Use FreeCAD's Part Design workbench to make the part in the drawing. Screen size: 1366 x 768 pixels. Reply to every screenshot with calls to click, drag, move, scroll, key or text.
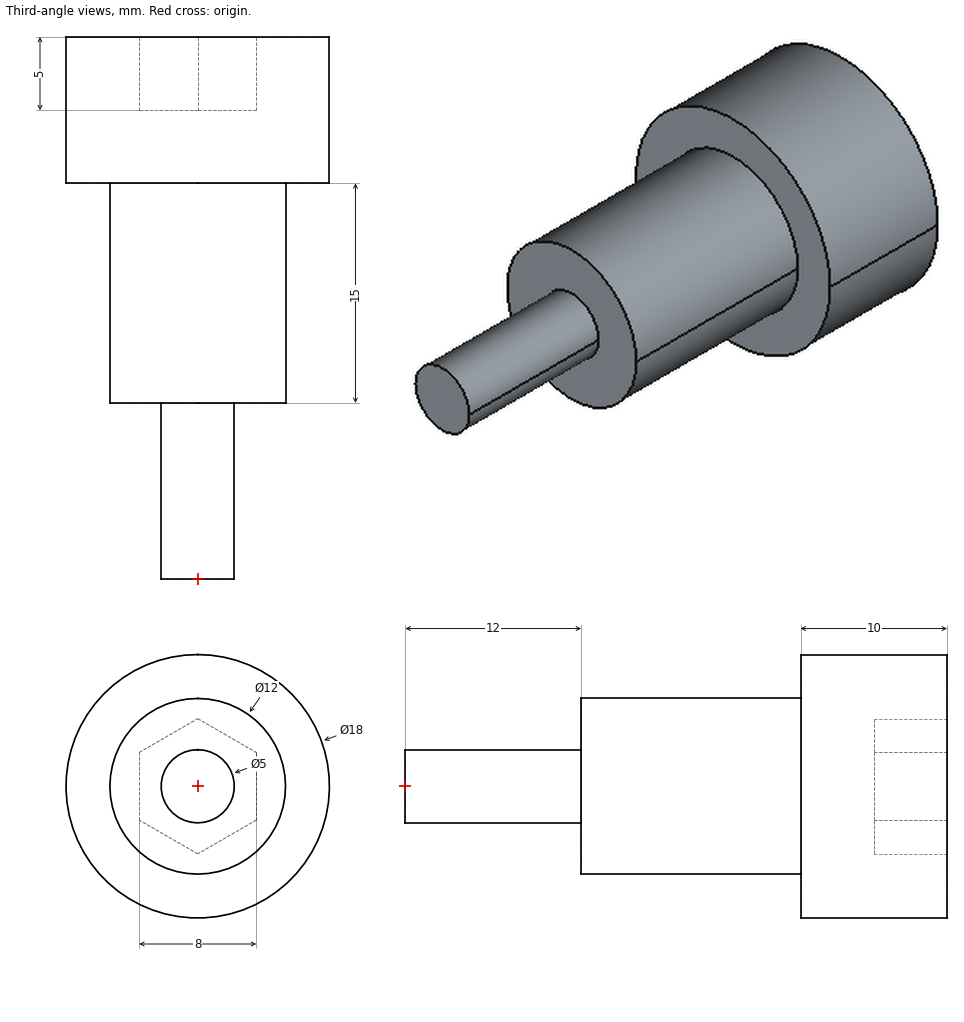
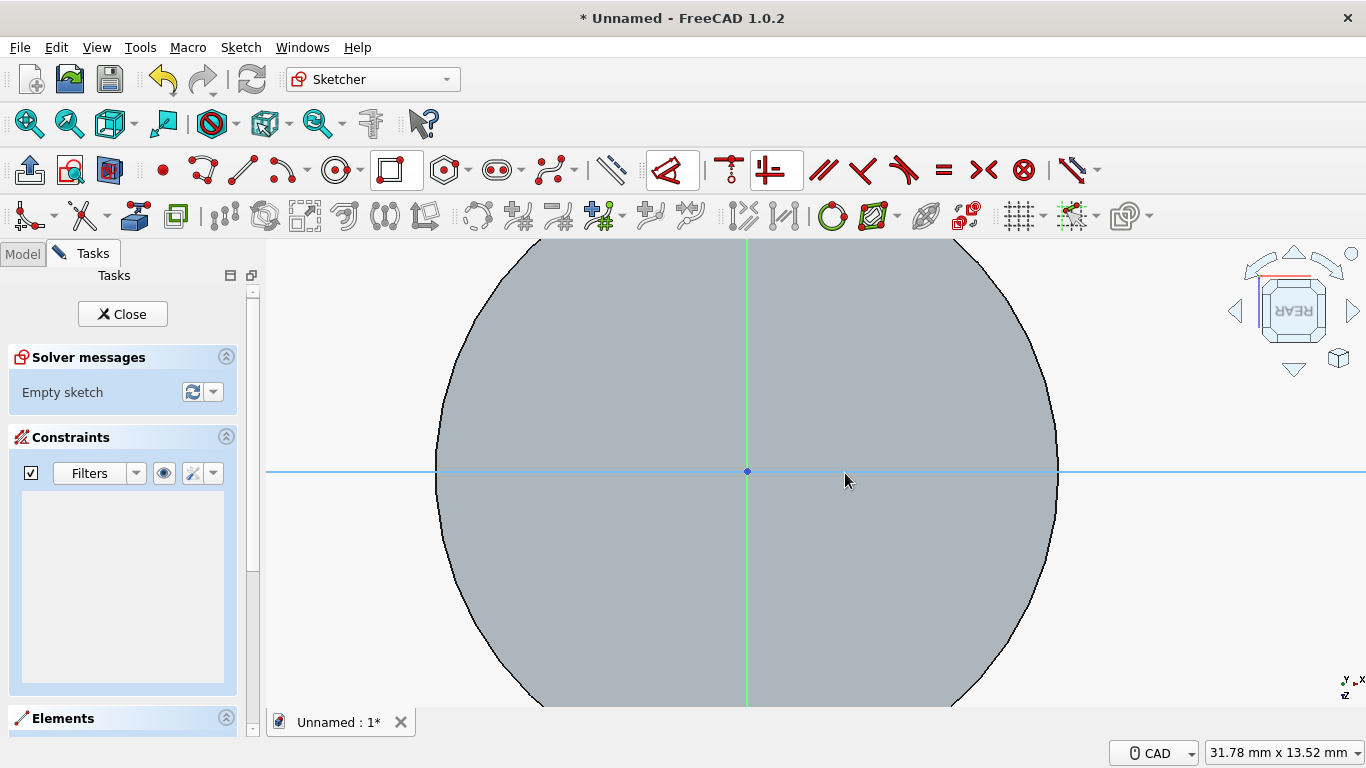
click(444, 170)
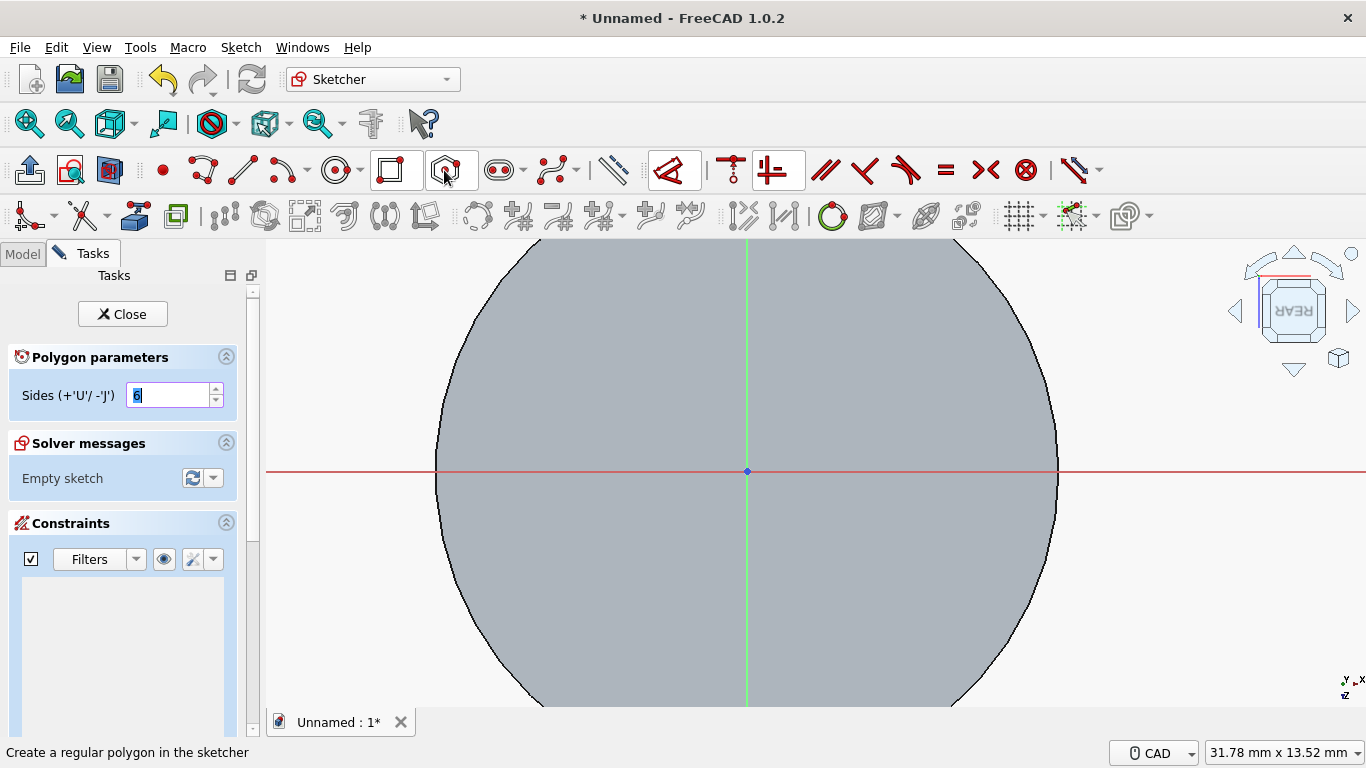
click(747, 472)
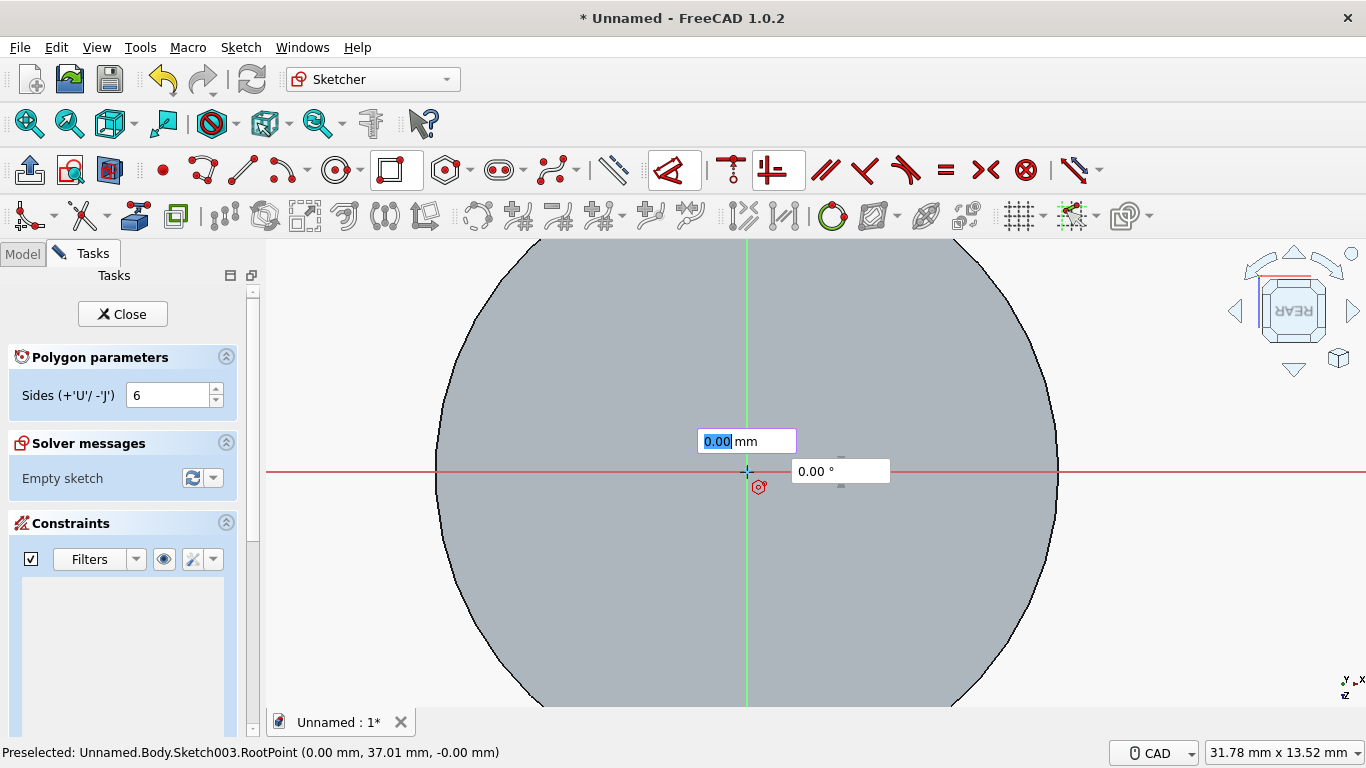
click(747, 312)
right_click(747, 312)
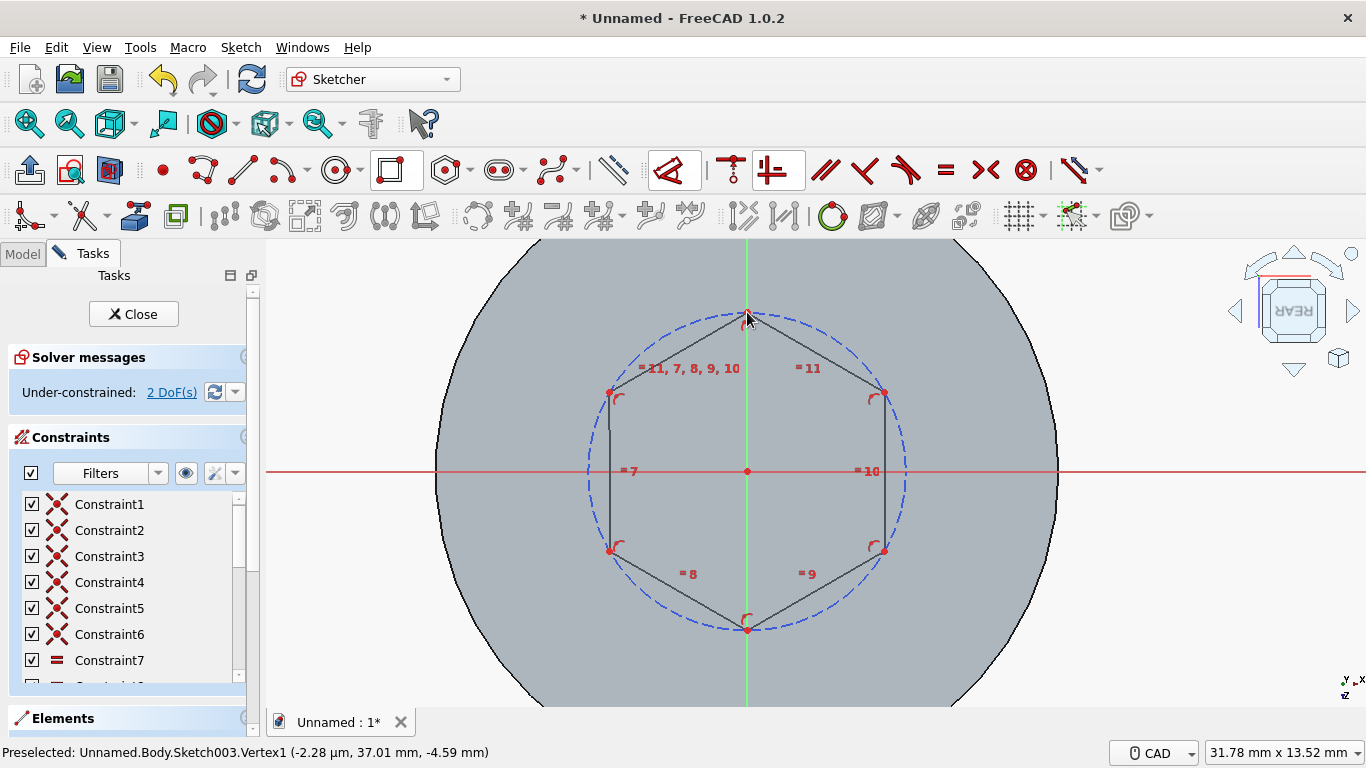
click(610, 440)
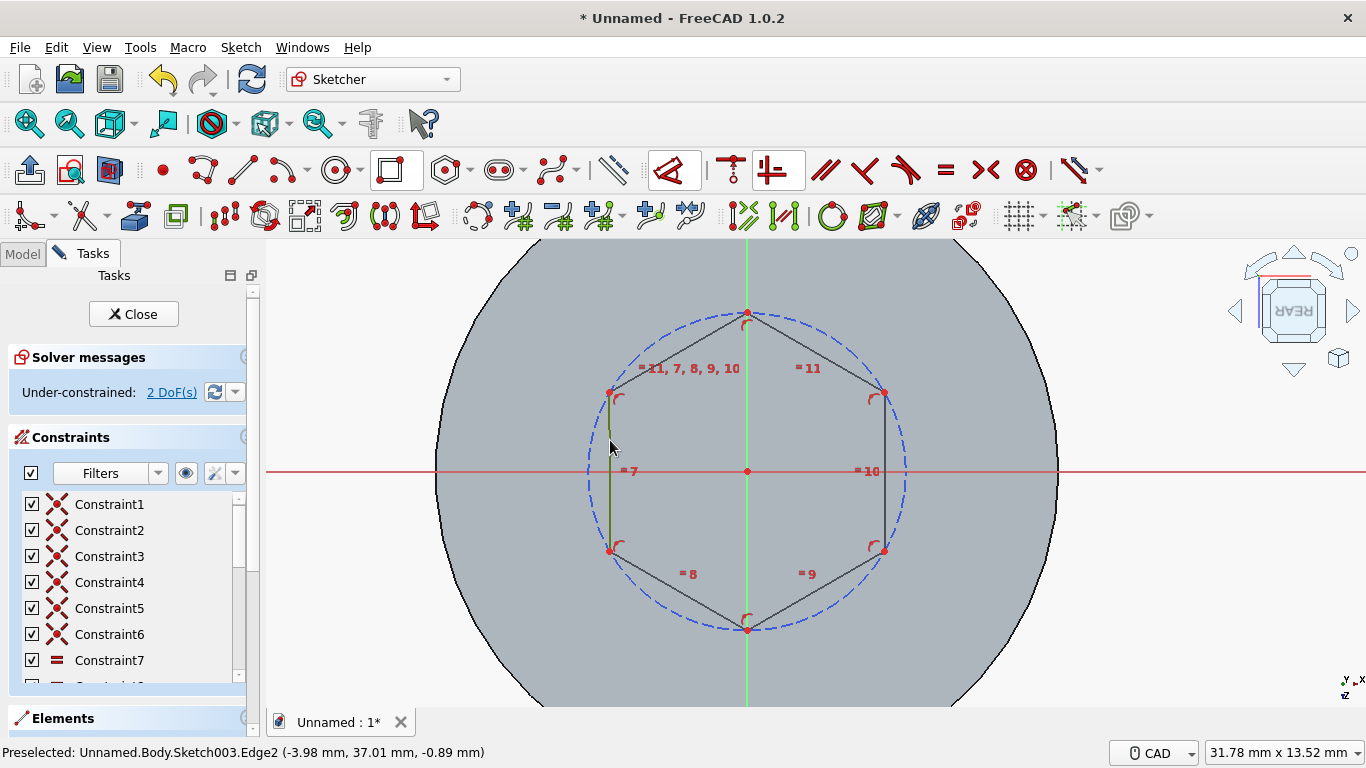
click(800, 170)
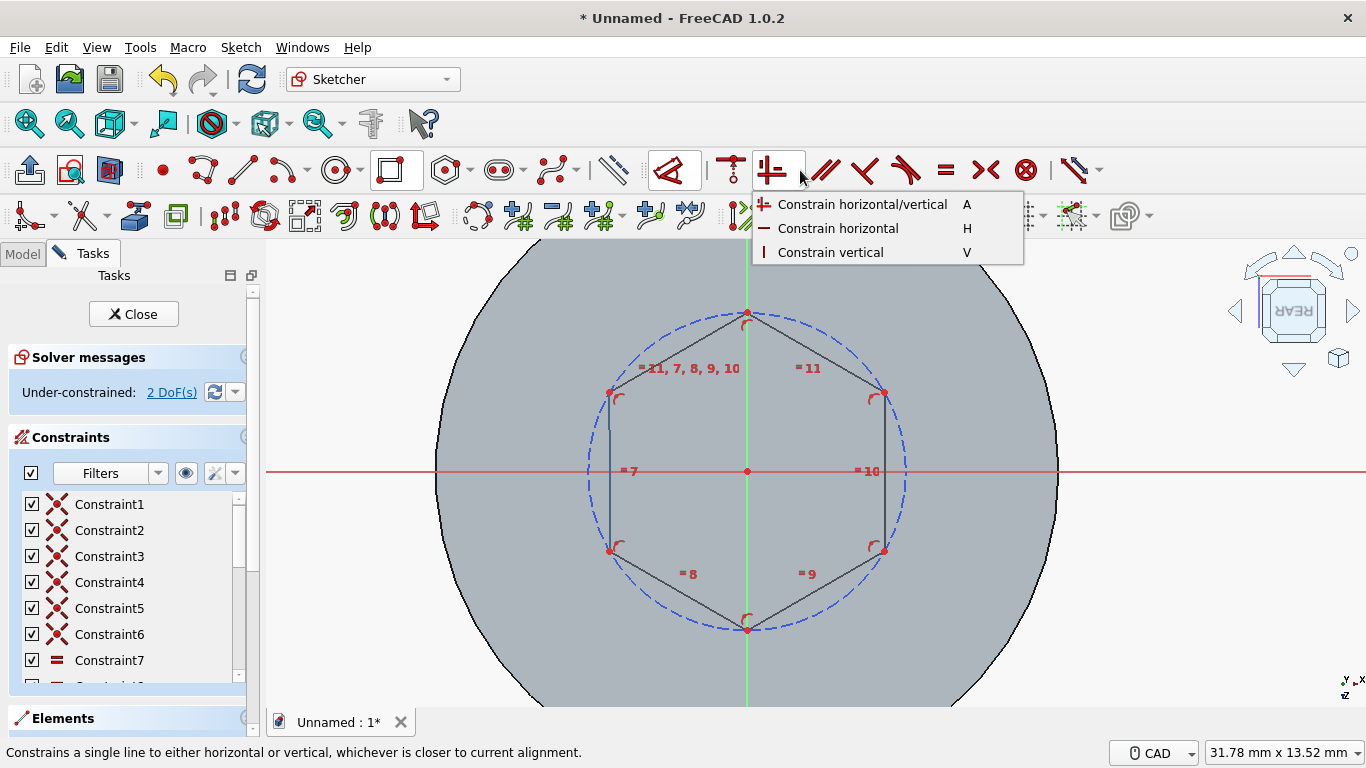
click(888, 252)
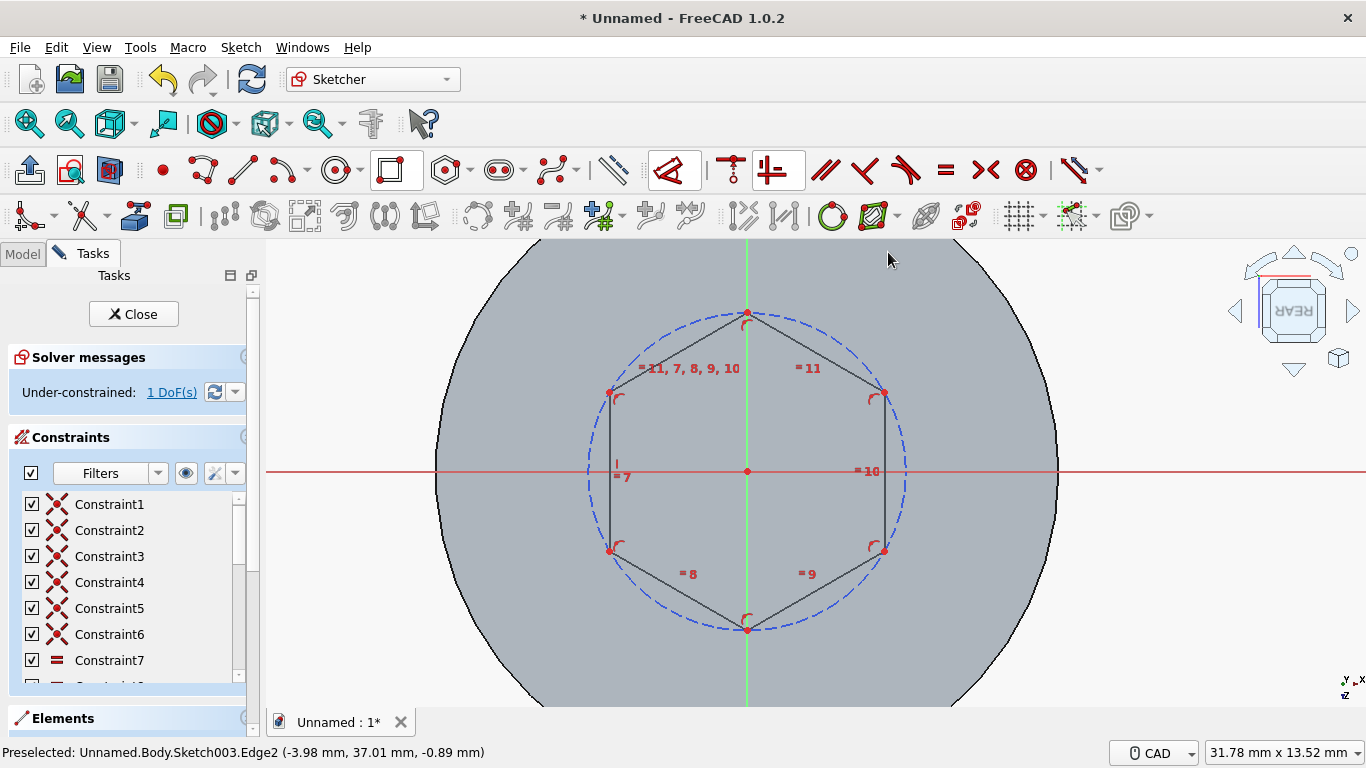
click(668, 170)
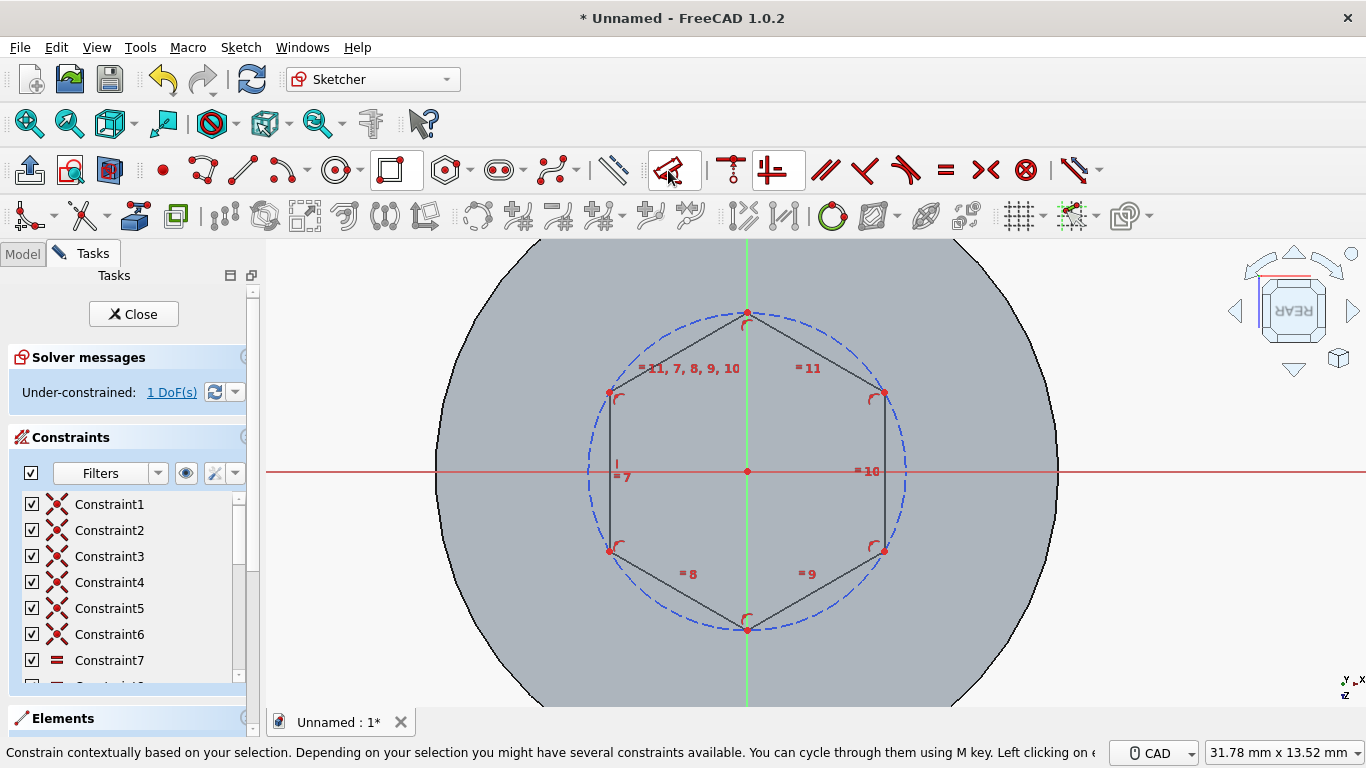
click(610, 392)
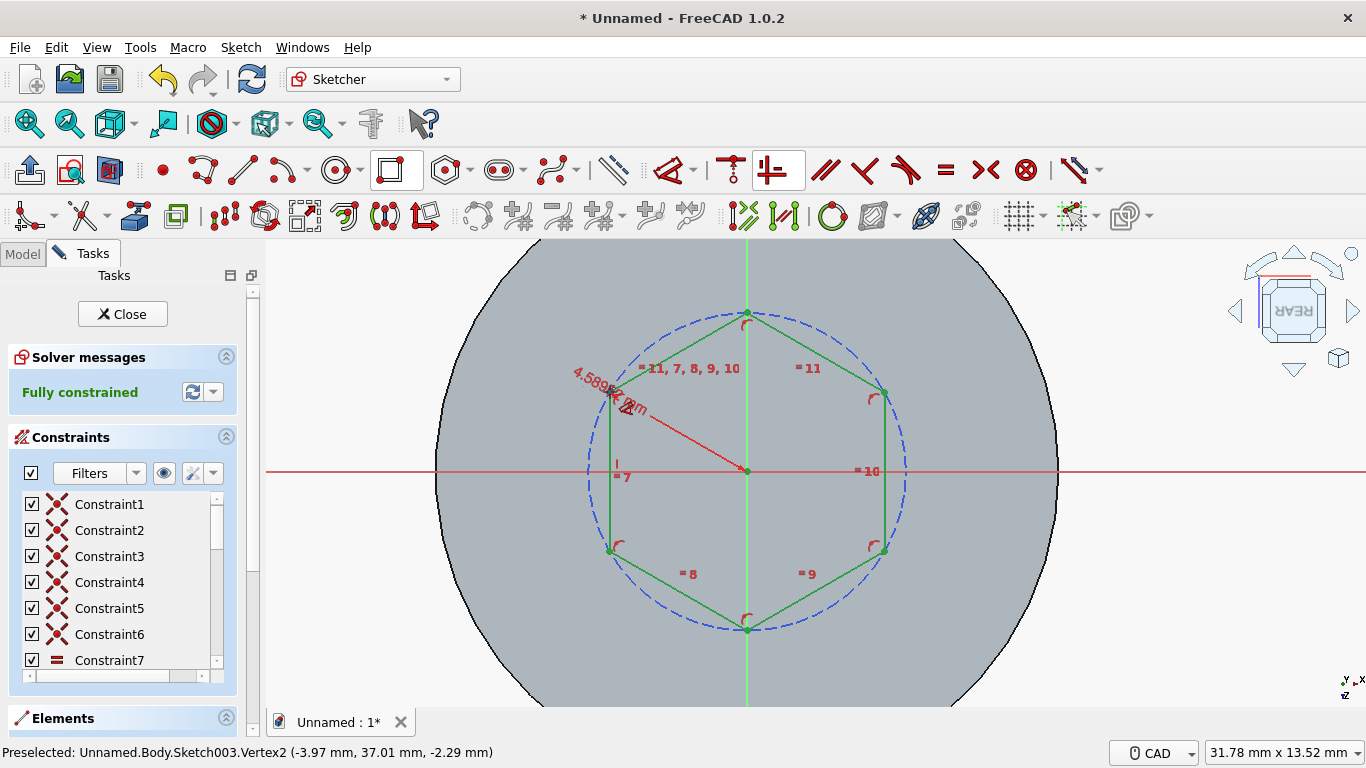
click(885, 551)
click(684, 310)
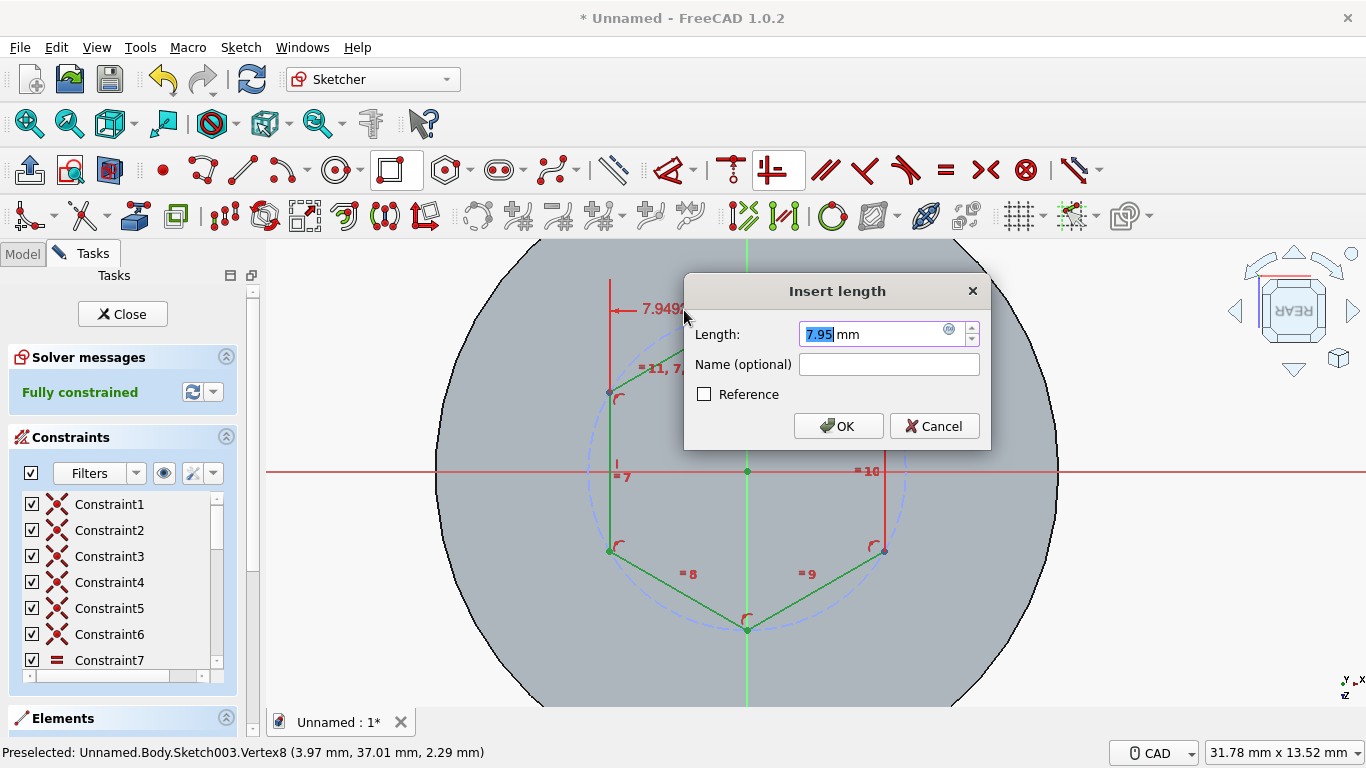
text(8)
key(Return)
key(Escape)